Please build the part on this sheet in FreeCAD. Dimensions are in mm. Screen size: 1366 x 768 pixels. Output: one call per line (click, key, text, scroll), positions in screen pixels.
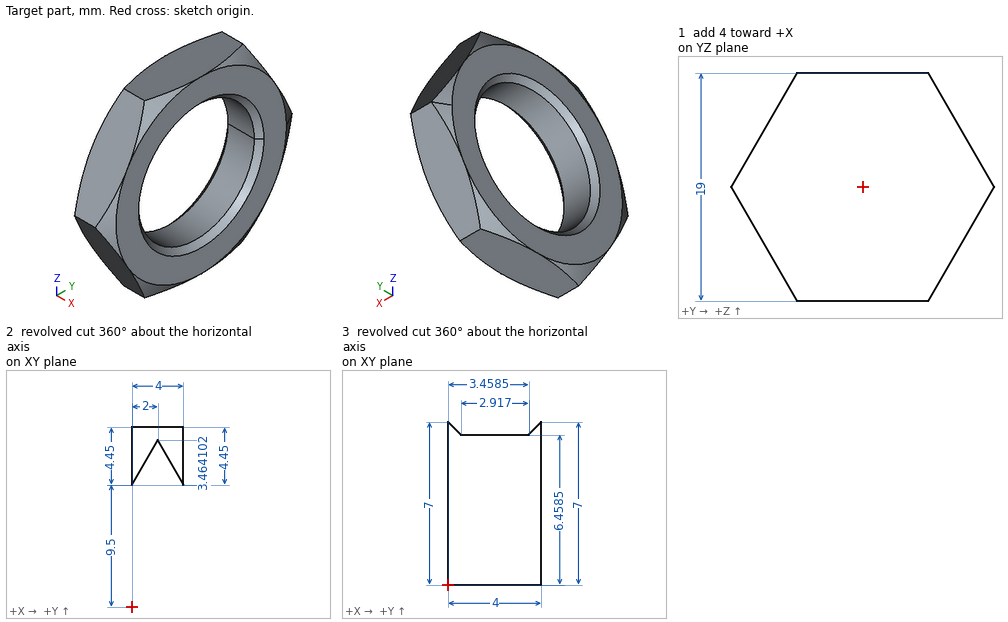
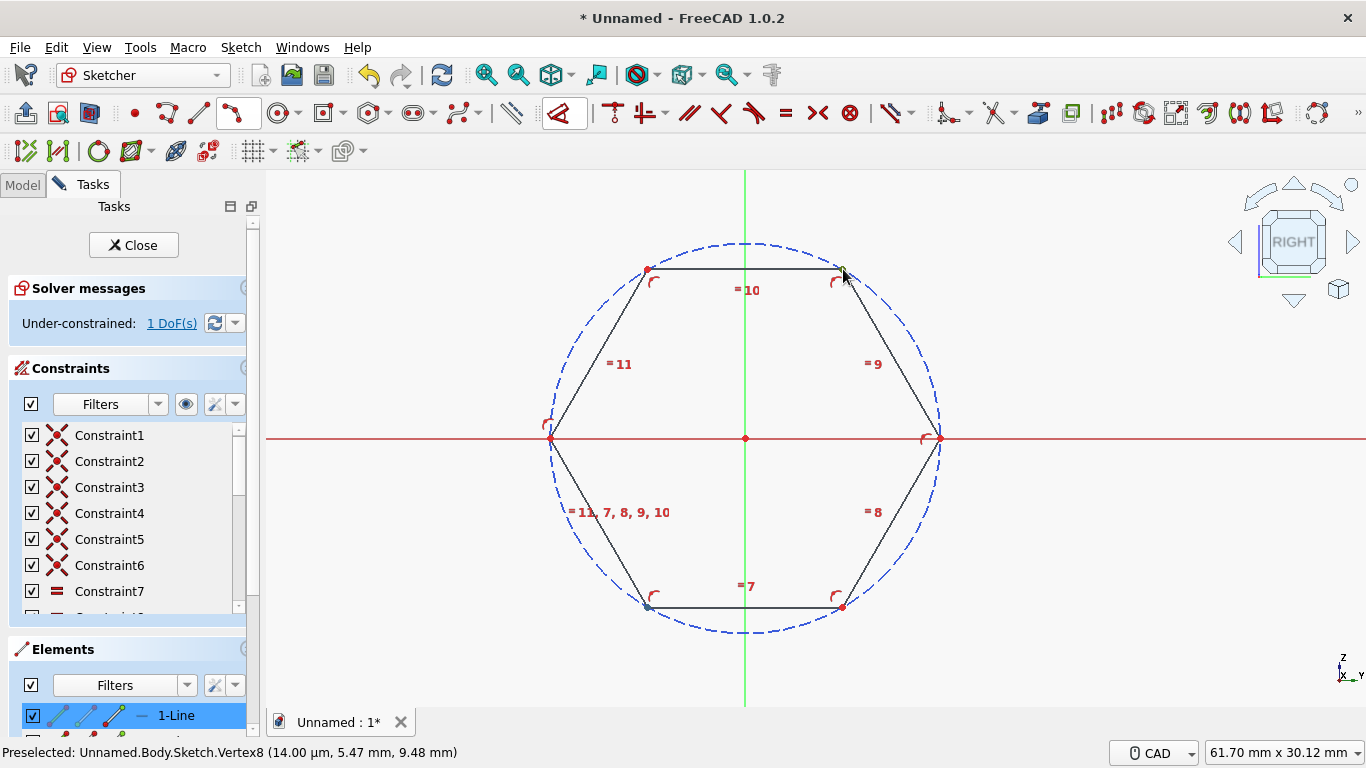
key(i)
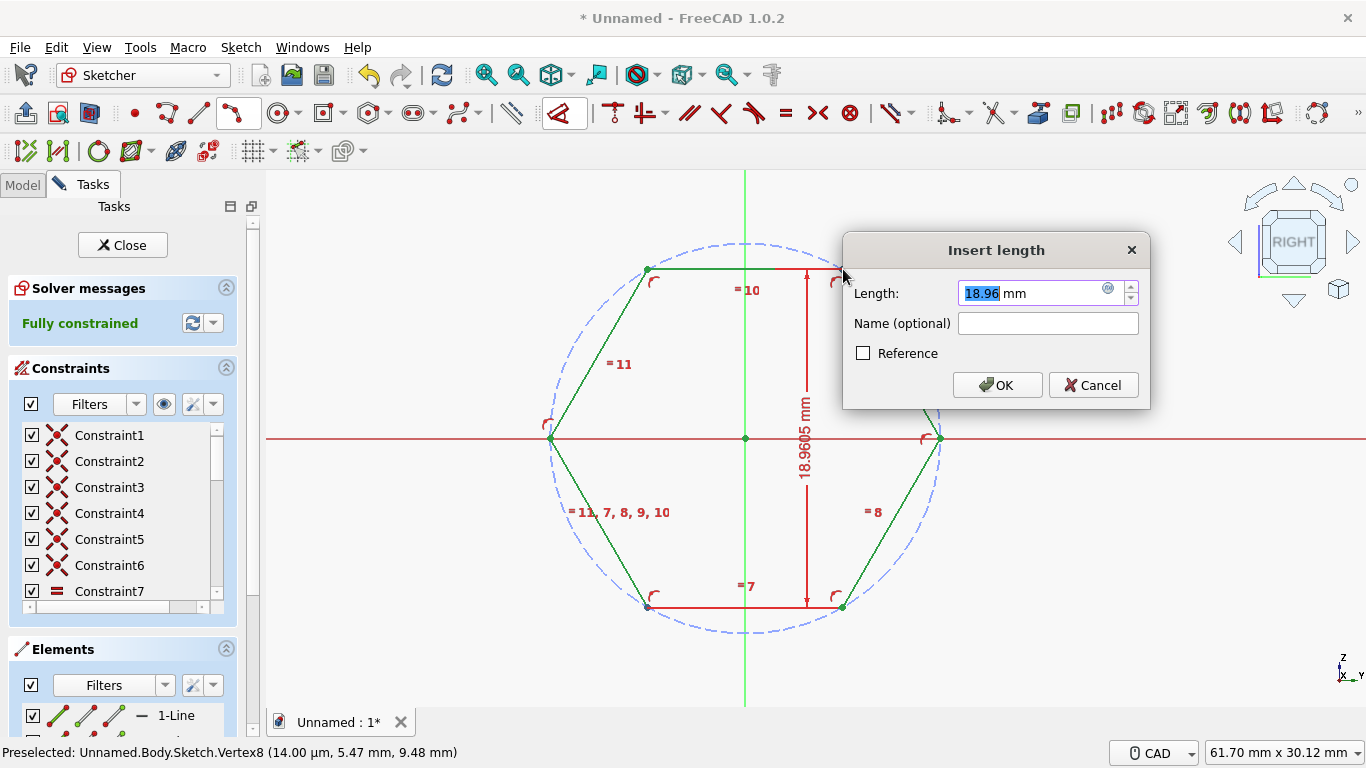
text(19)
key(Return)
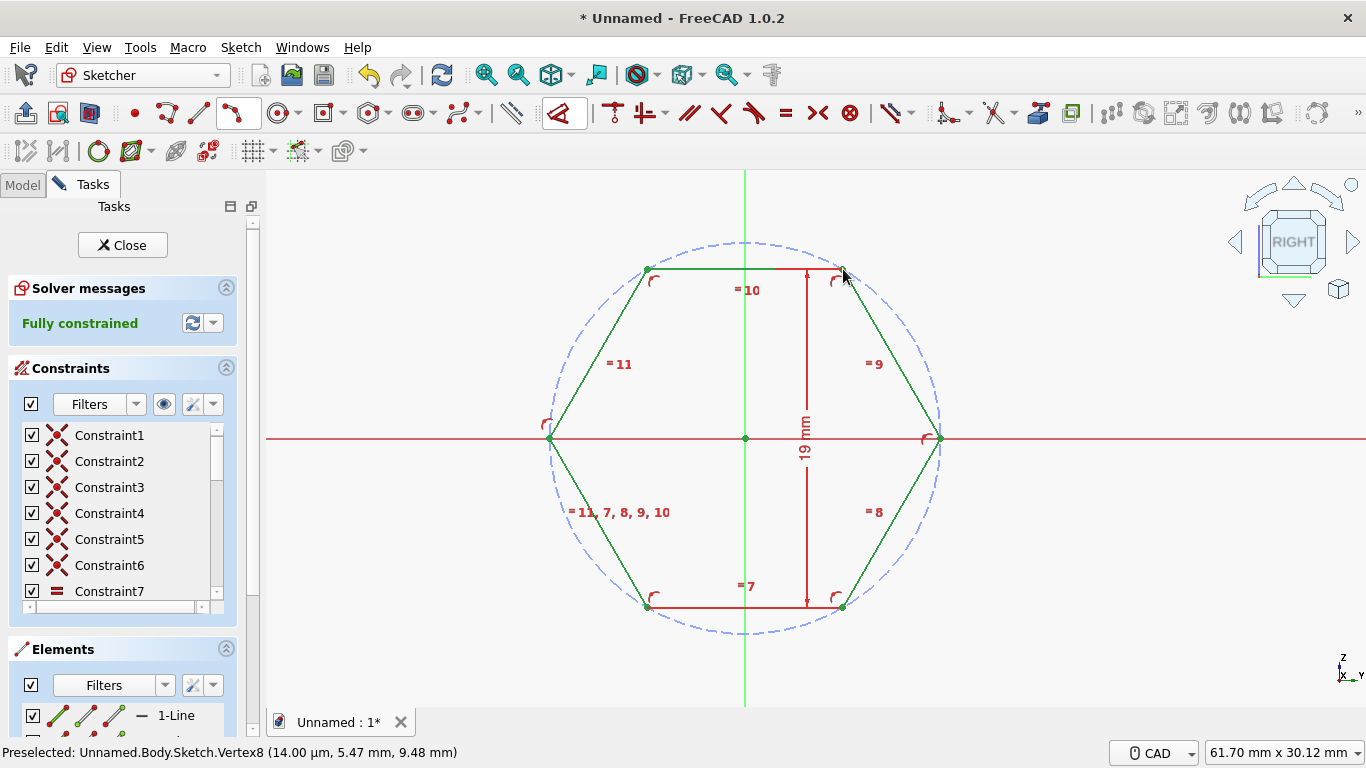
click(123, 245)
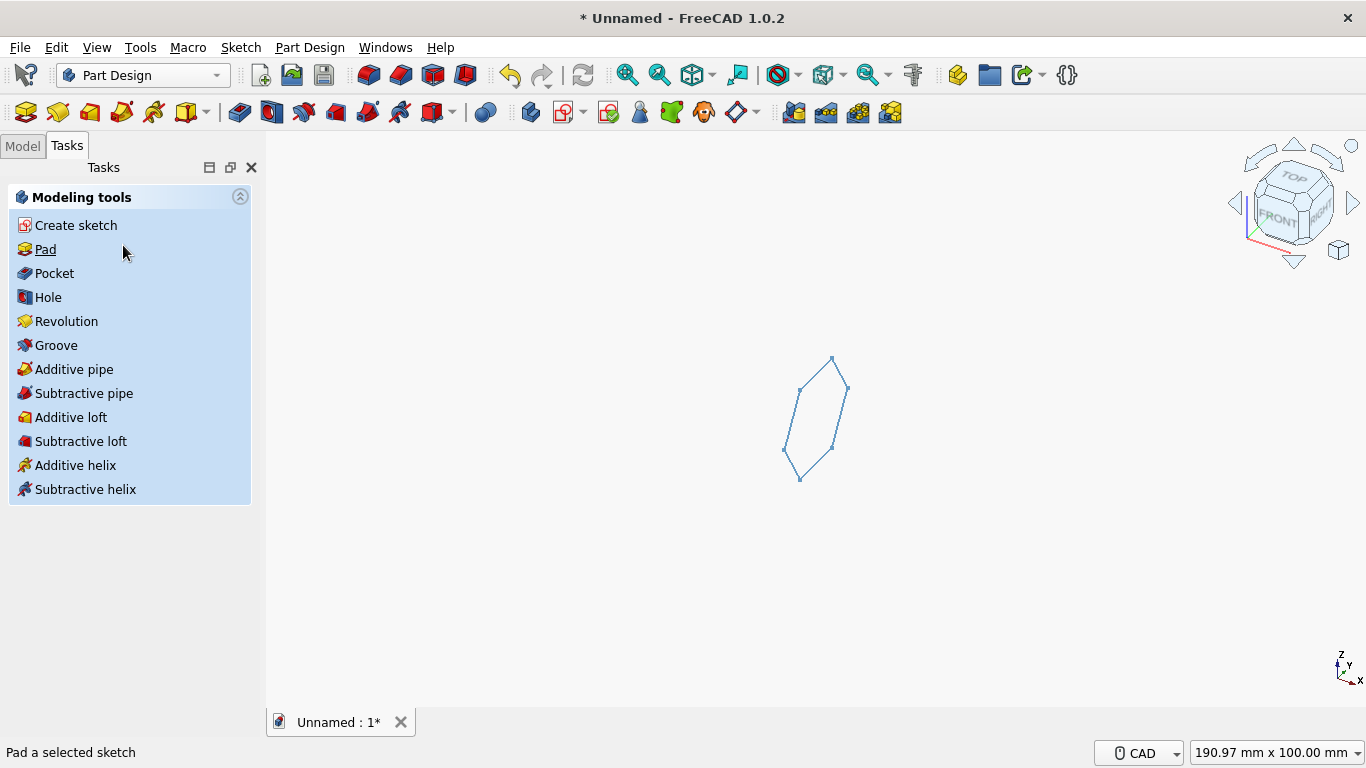
click(26, 112)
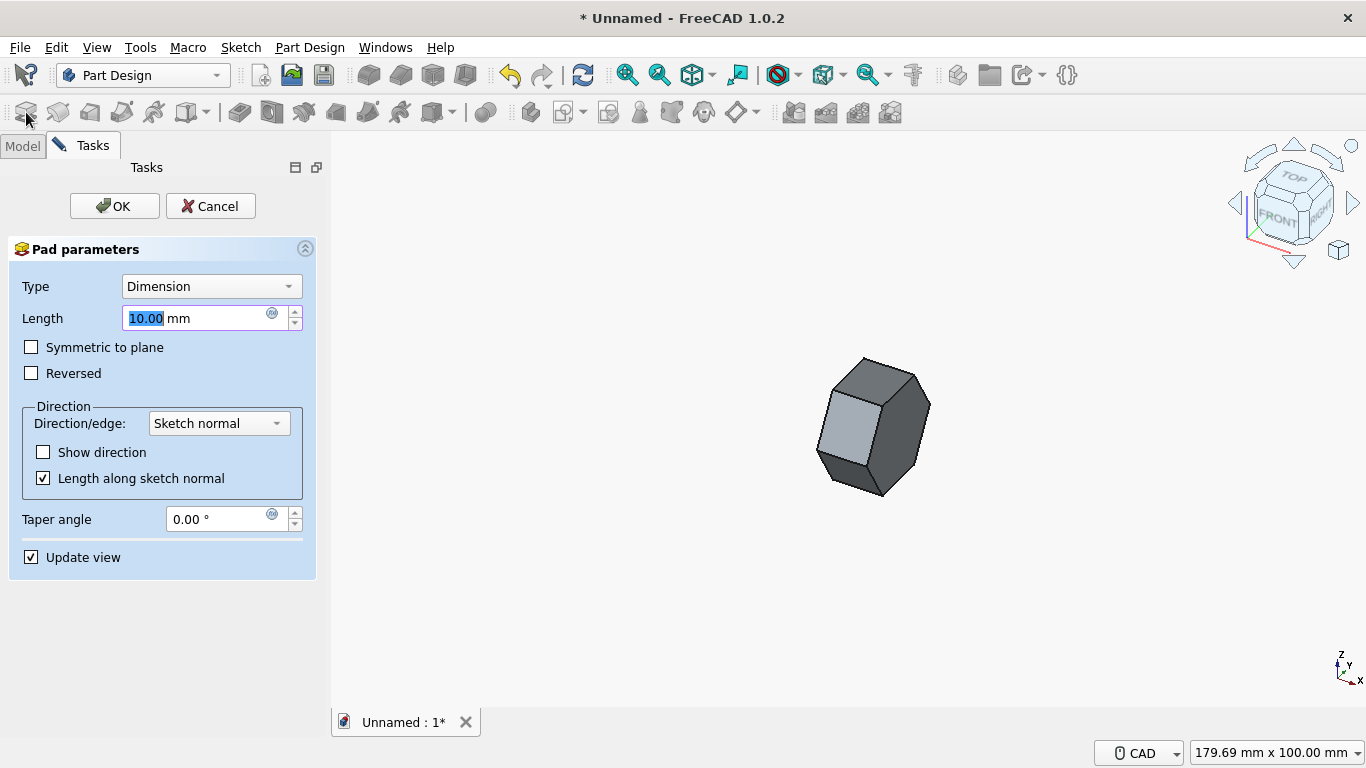
text(4)
key(Tab)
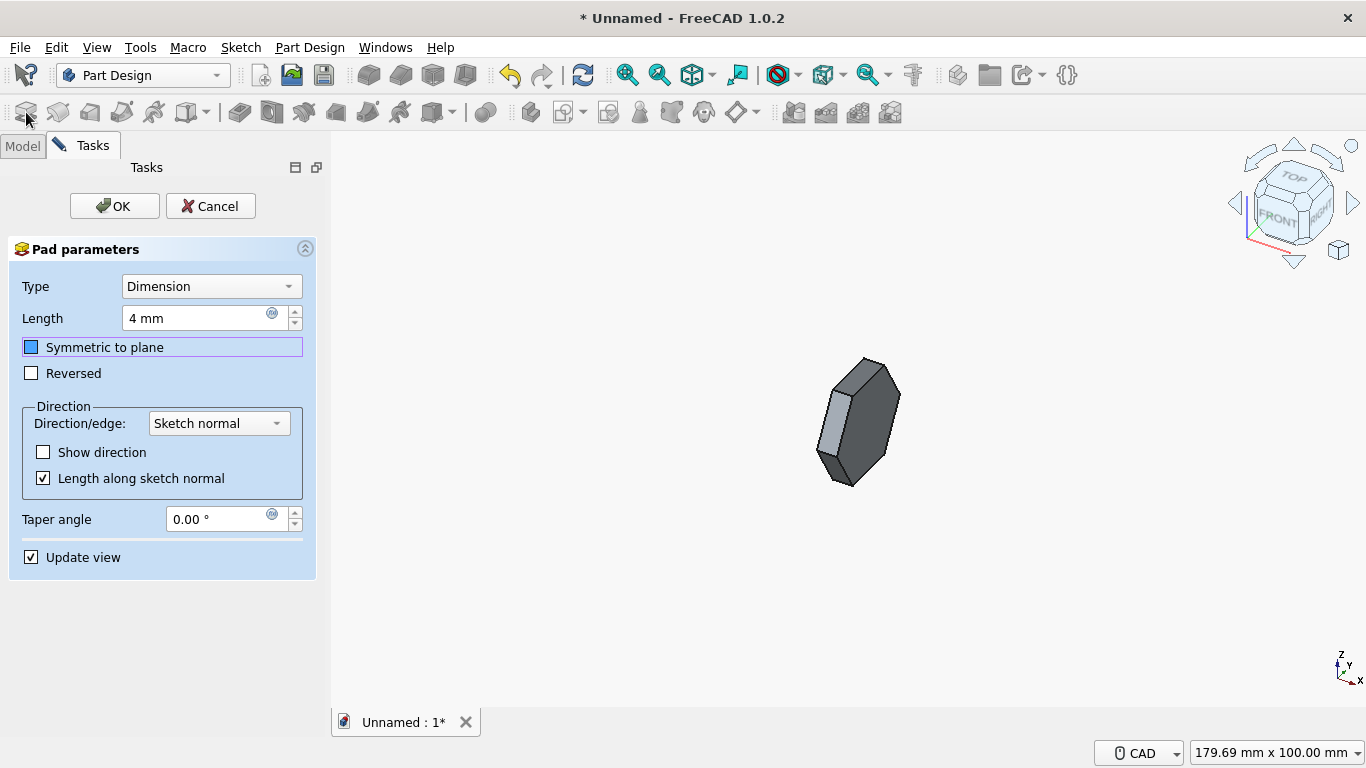
click(115, 206)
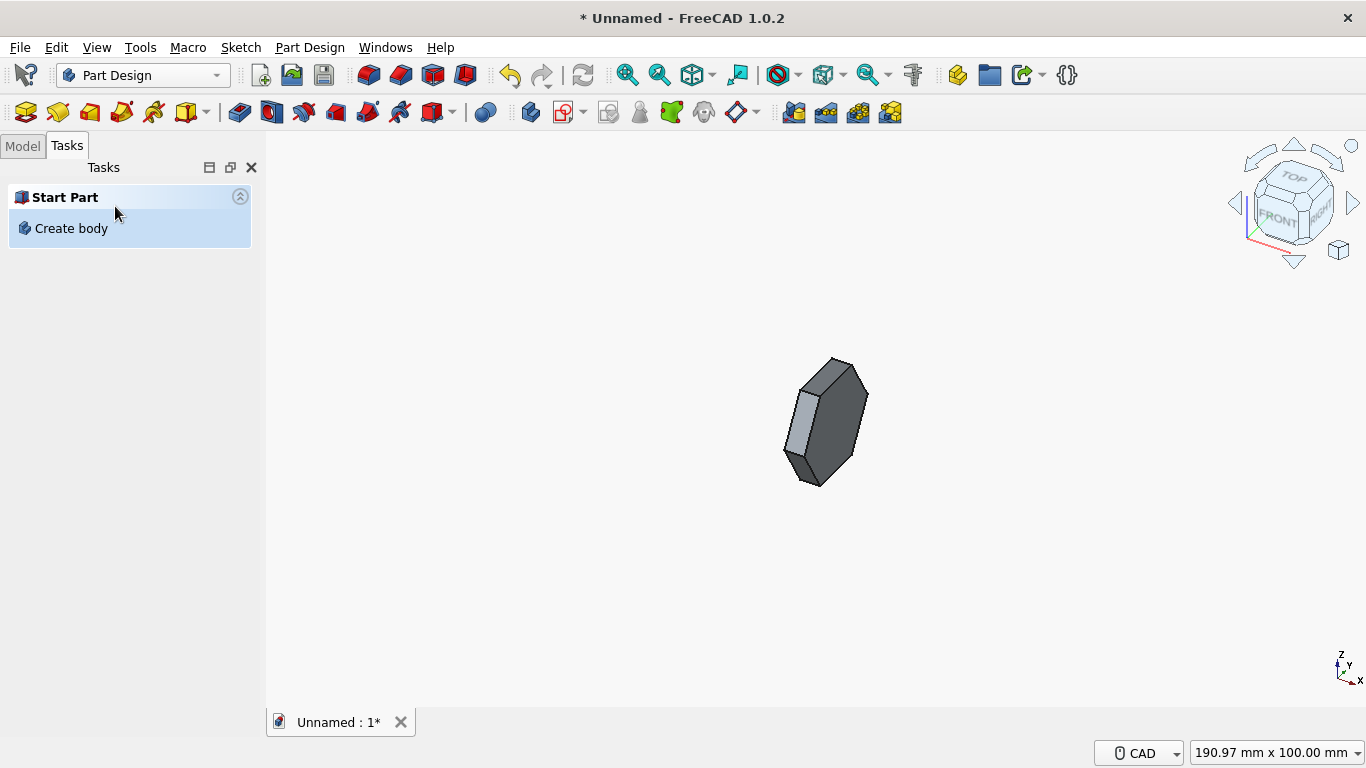
click(628, 76)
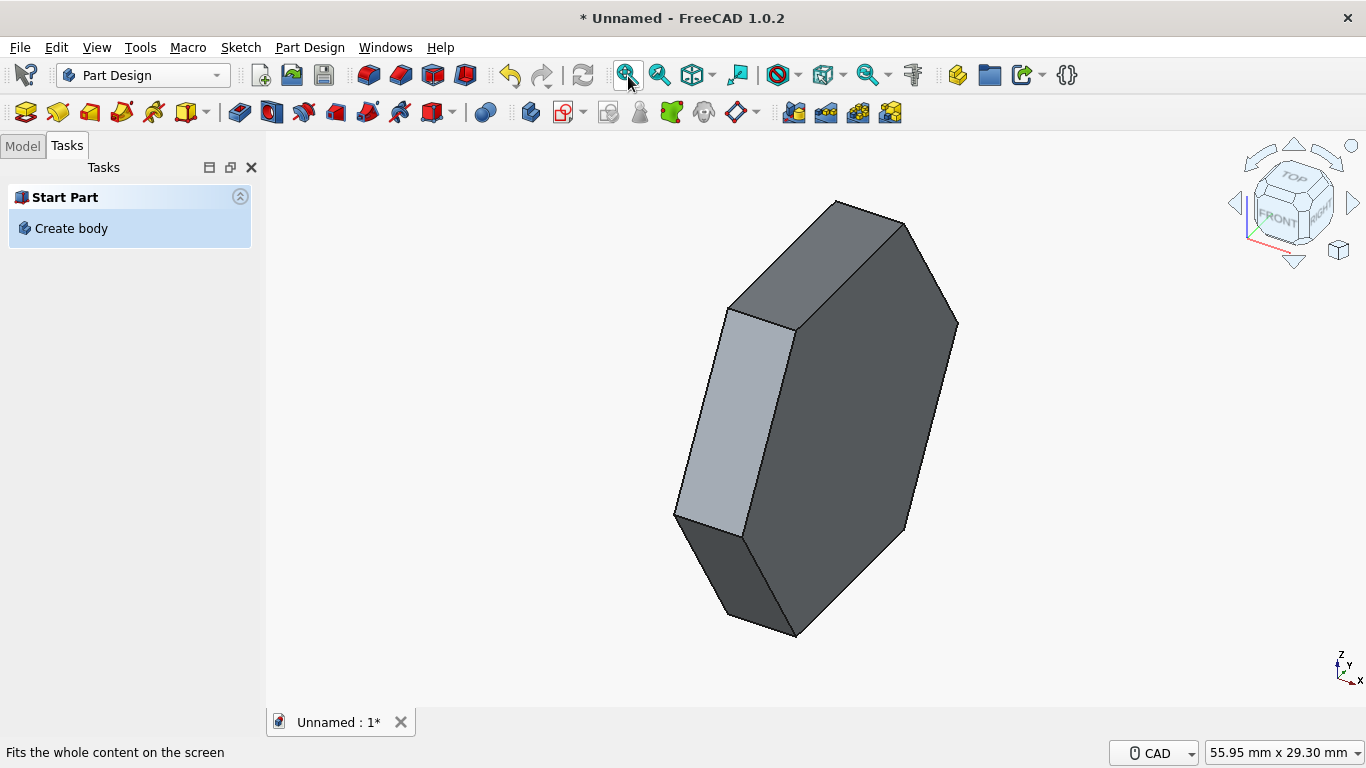
click(564, 112)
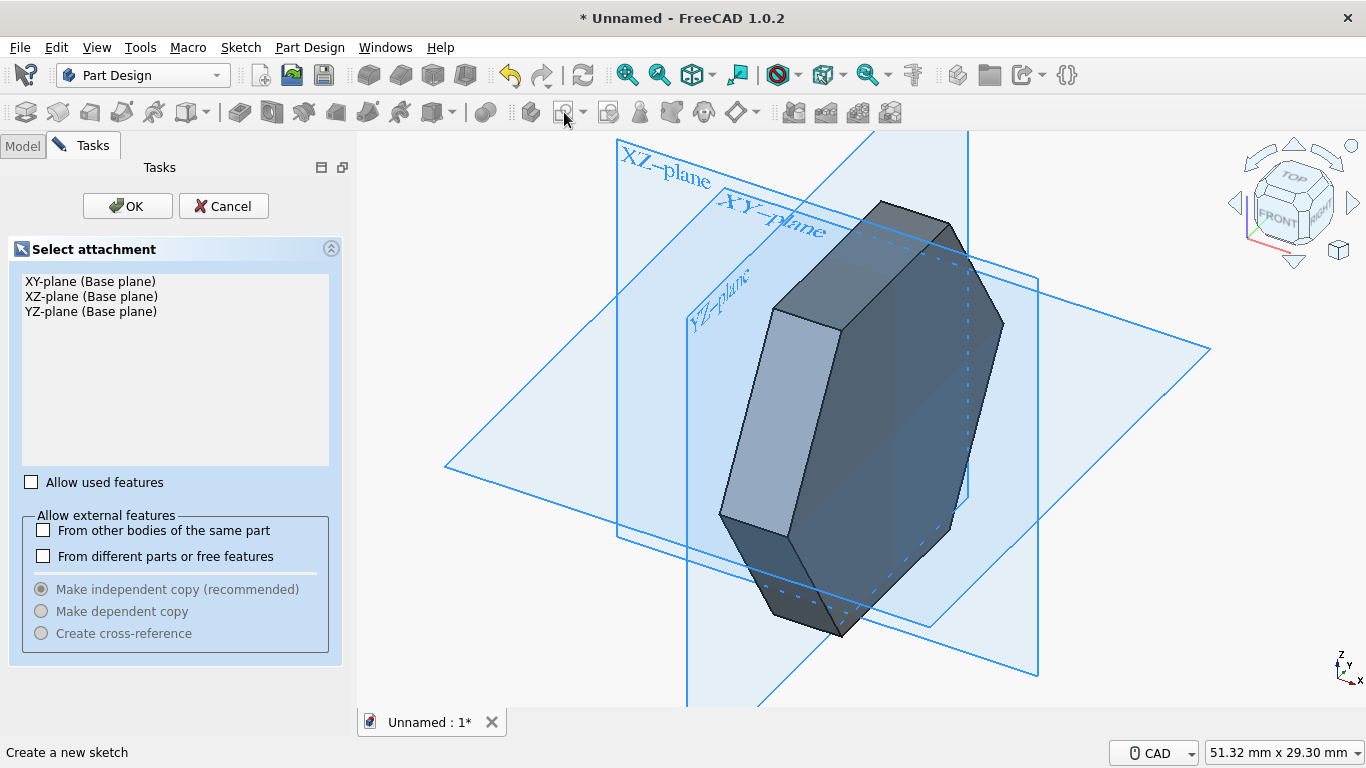
click(82, 282)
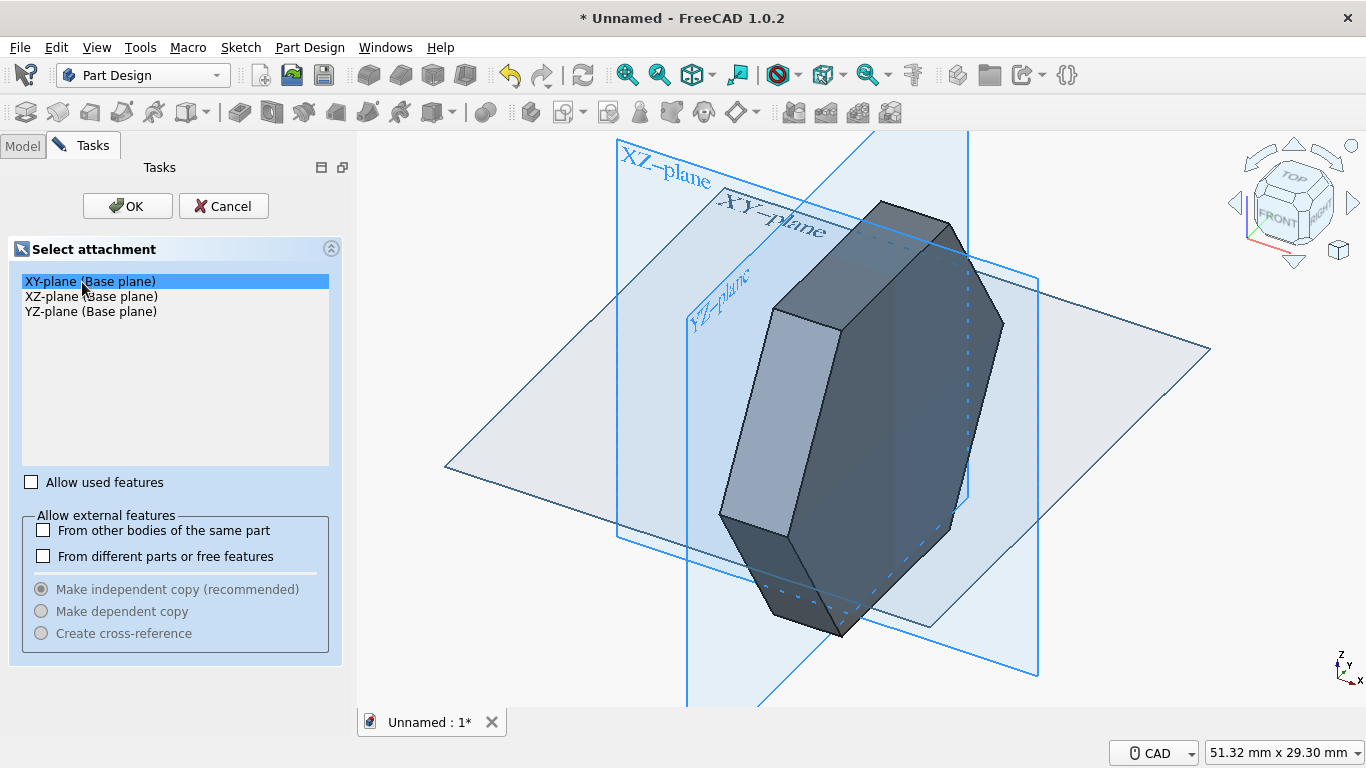
click(128, 206)